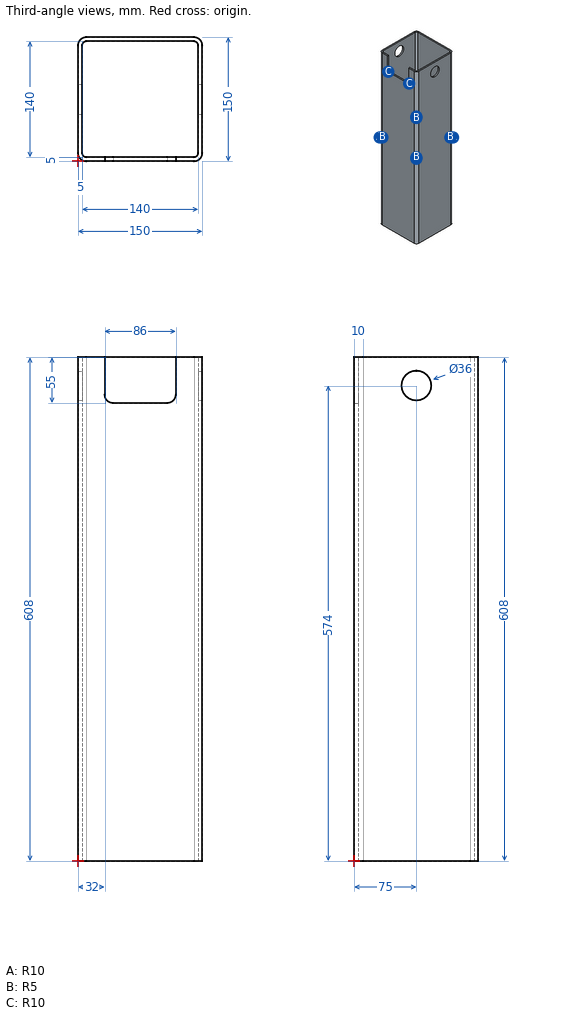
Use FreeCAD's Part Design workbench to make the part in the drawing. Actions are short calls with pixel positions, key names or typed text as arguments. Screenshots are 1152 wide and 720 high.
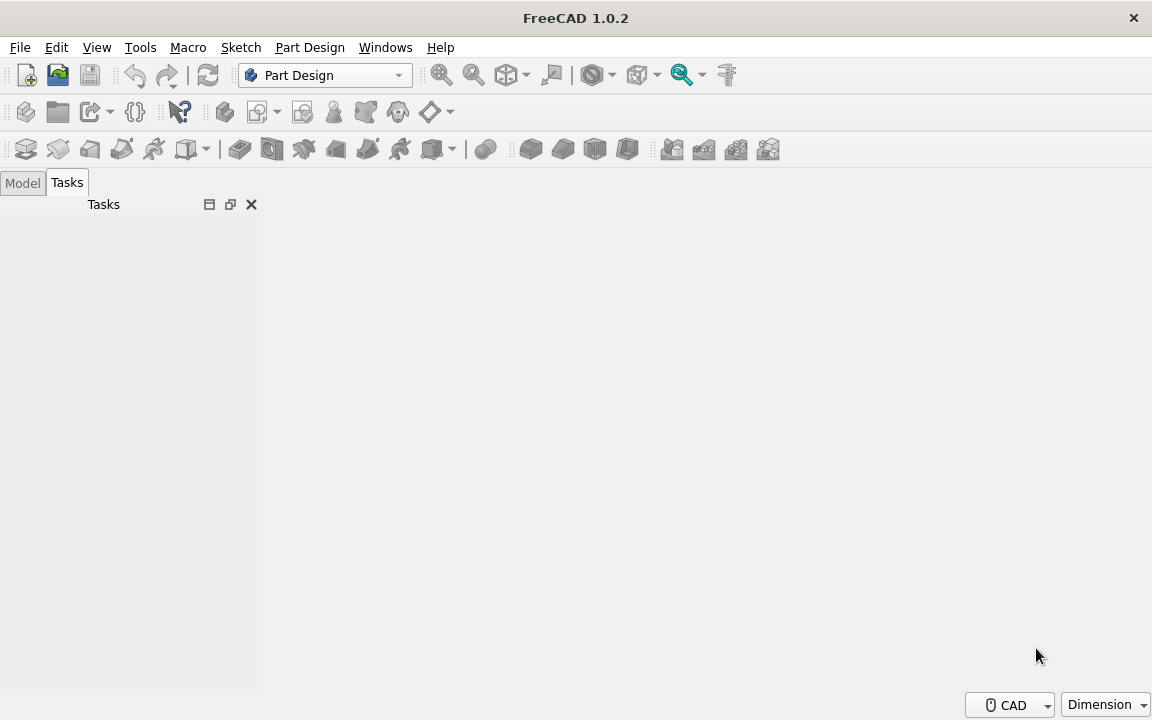
key(ctrl+n)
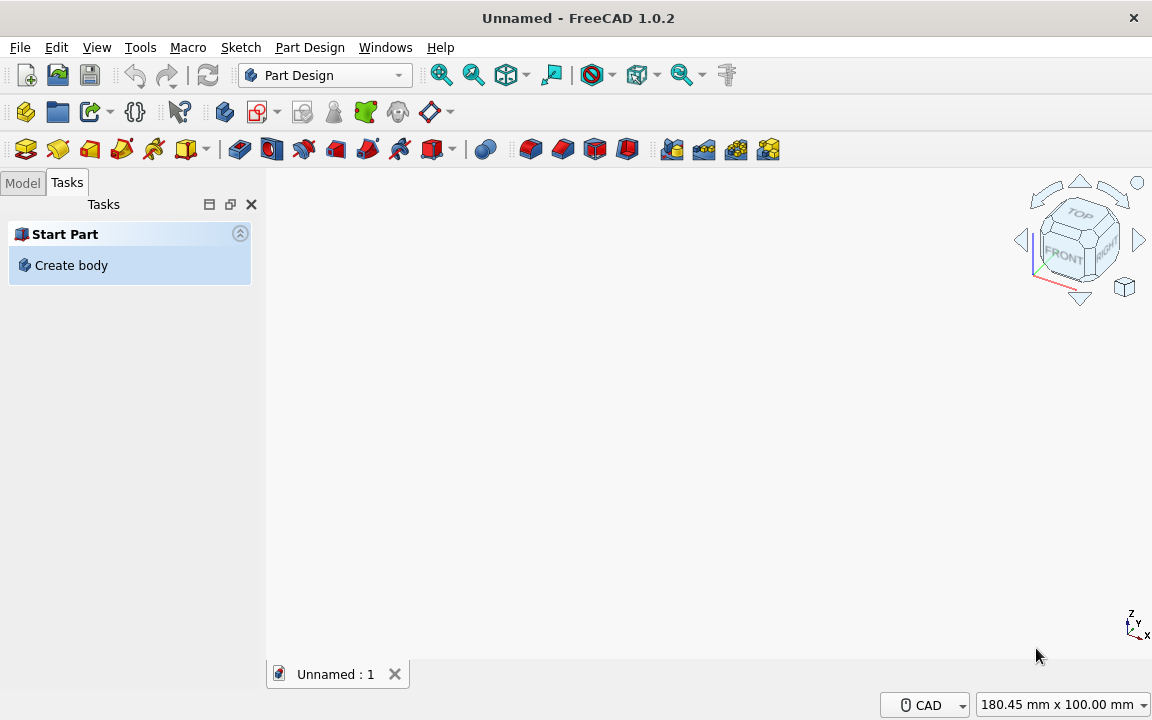
click(258, 112)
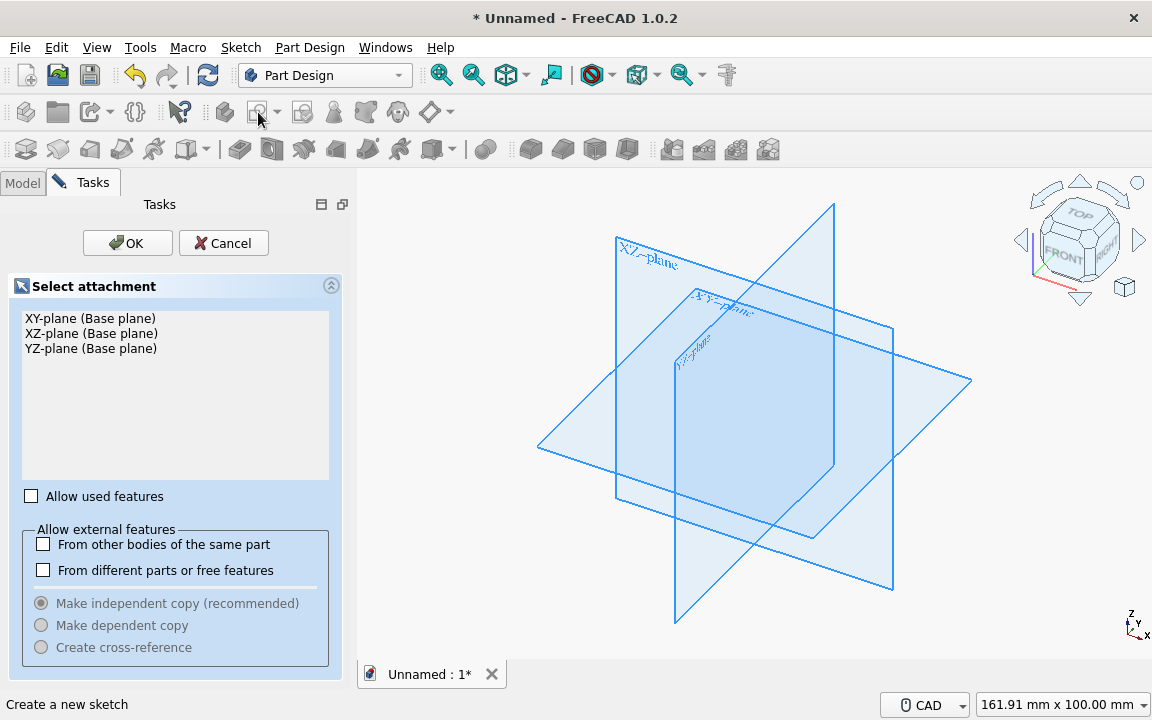
click(82, 318)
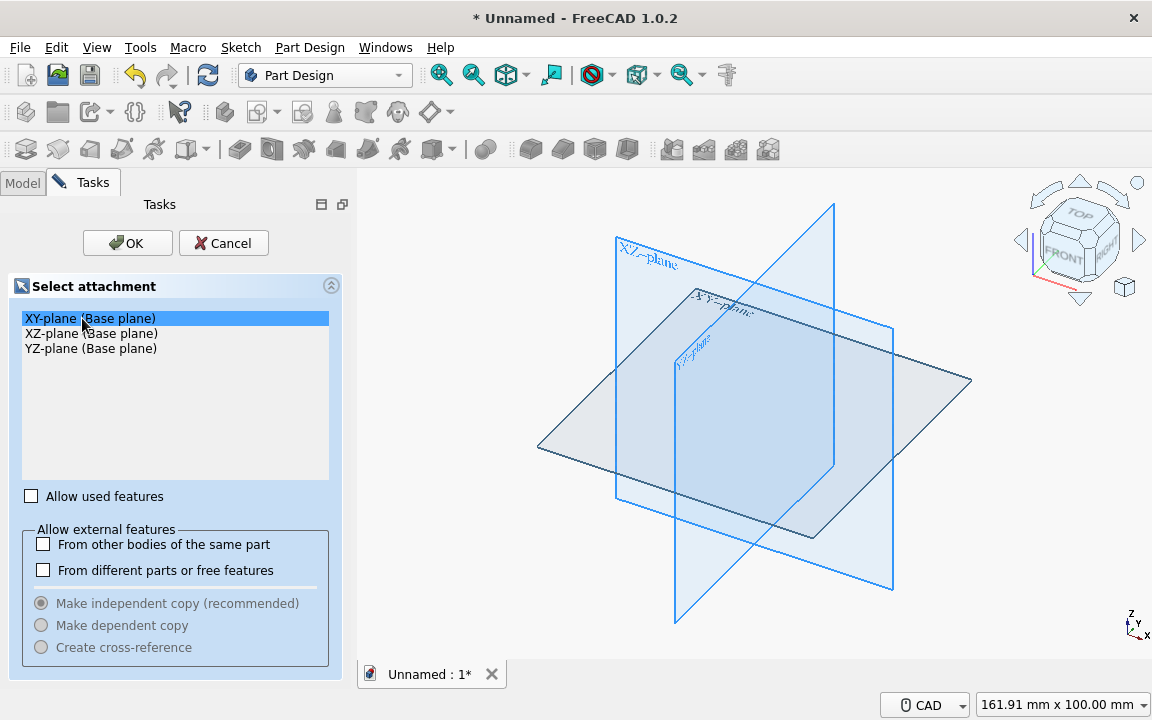
click(128, 243)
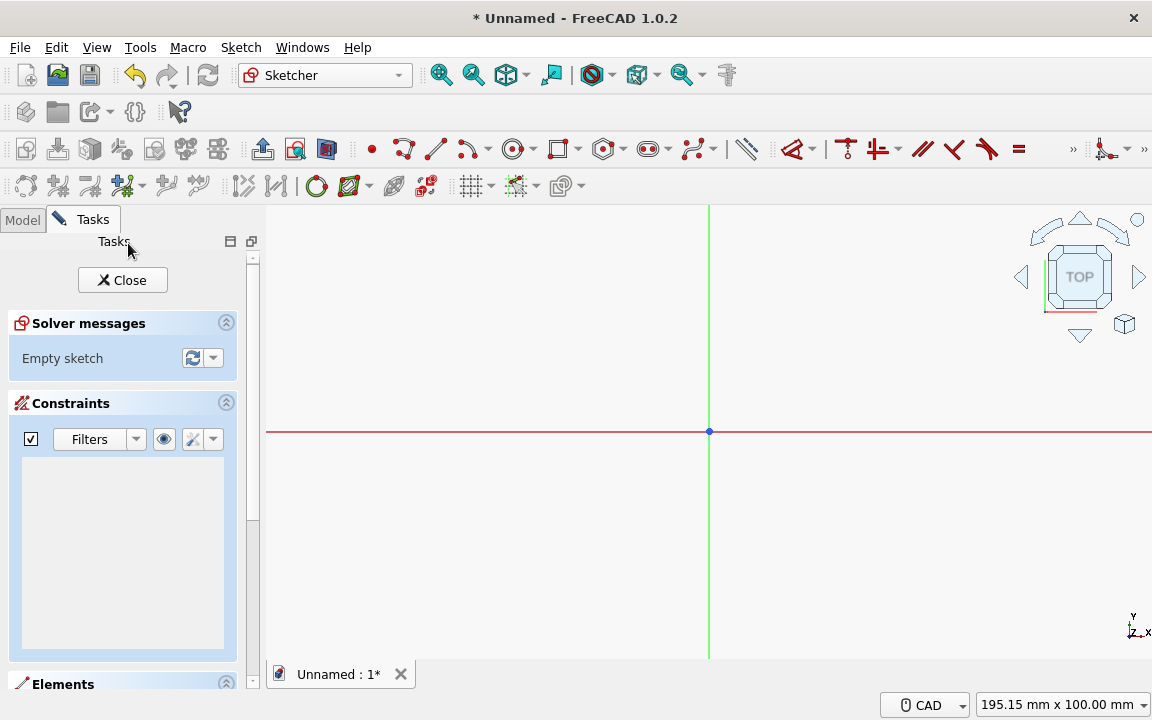
scroll(402, 630, down, 5)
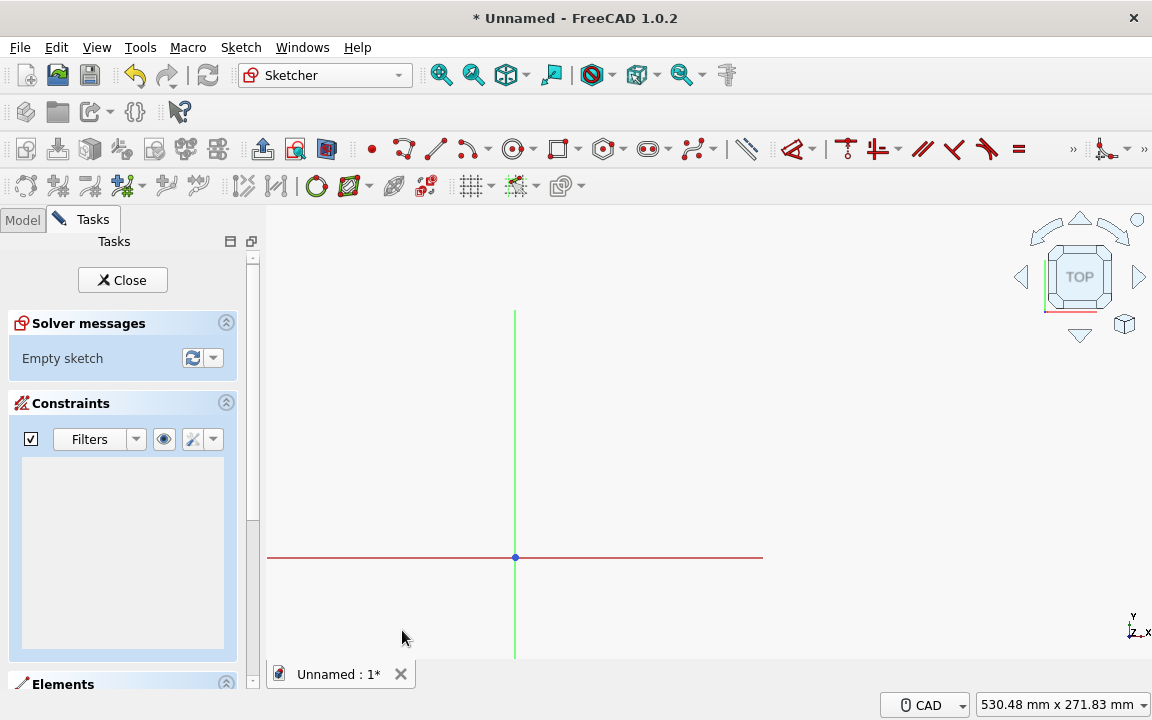
key(g)
key(r)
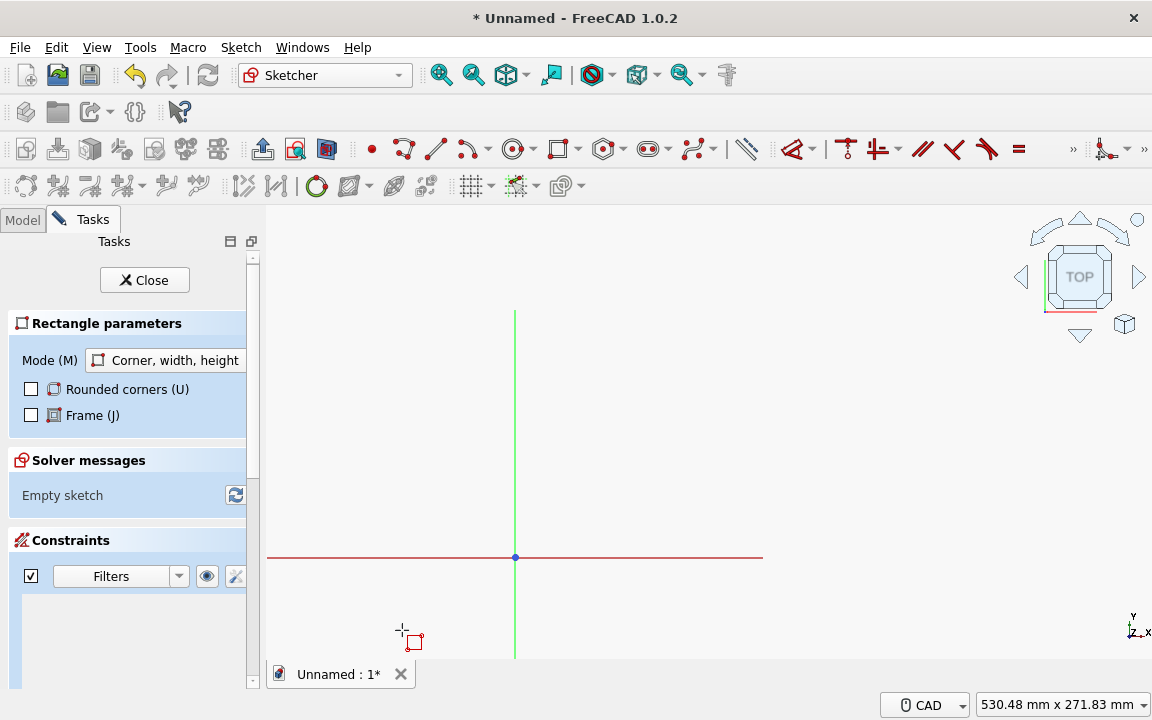
click(515, 558)
click(766, 307)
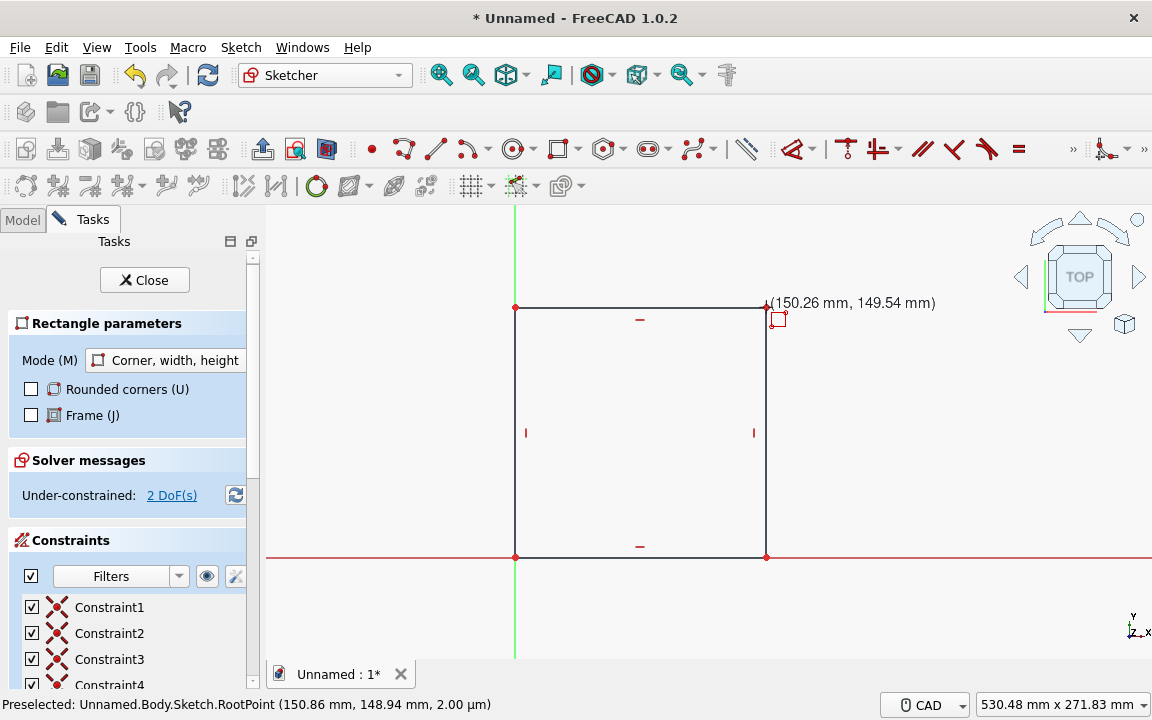
scroll(523, 316, up, 4)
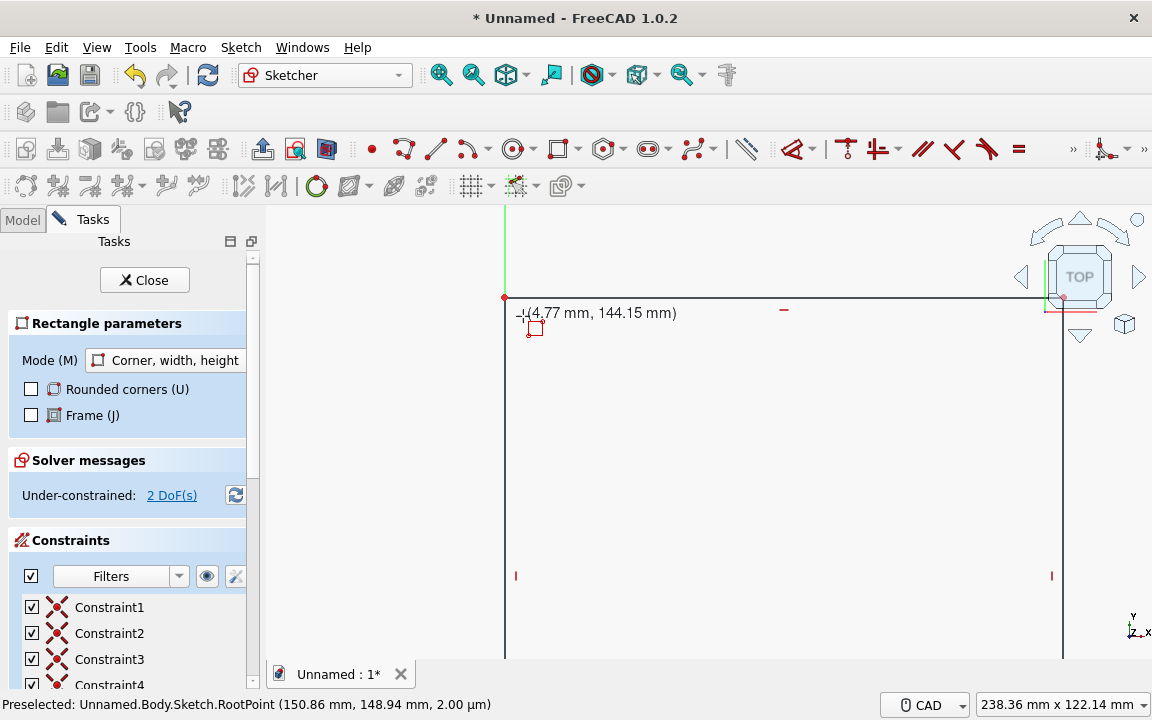
click(524, 315)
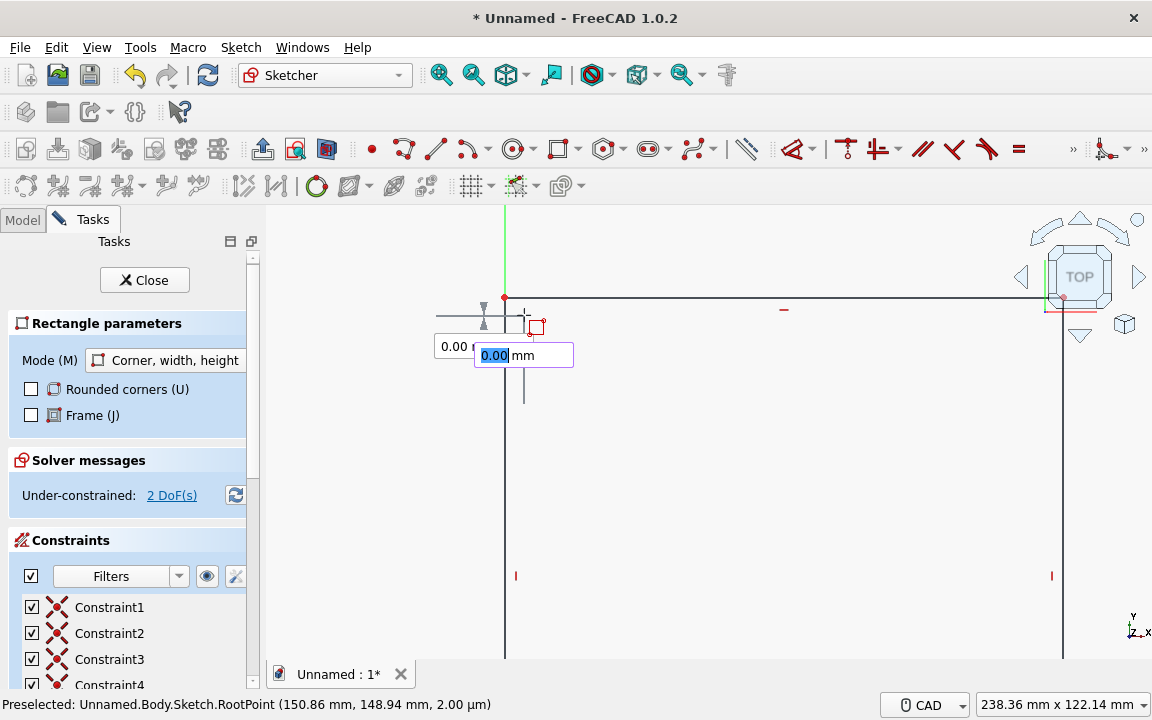
scroll(466, 258, down, 3)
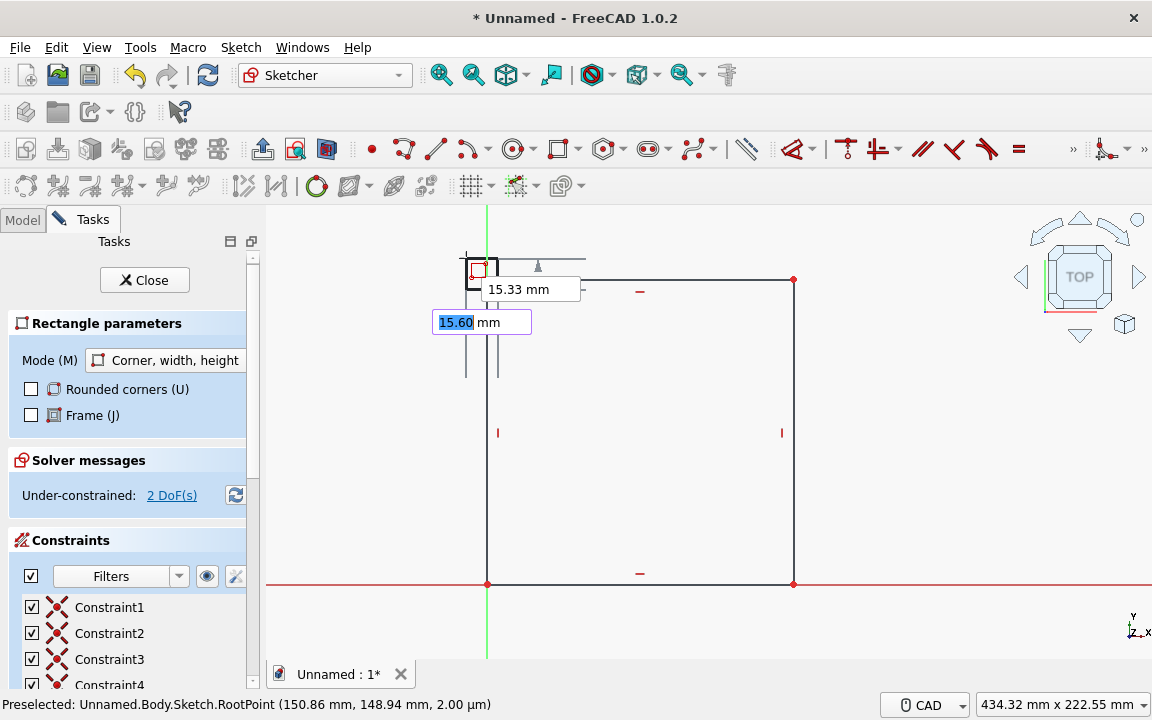
scroll(783, 575, up, 3)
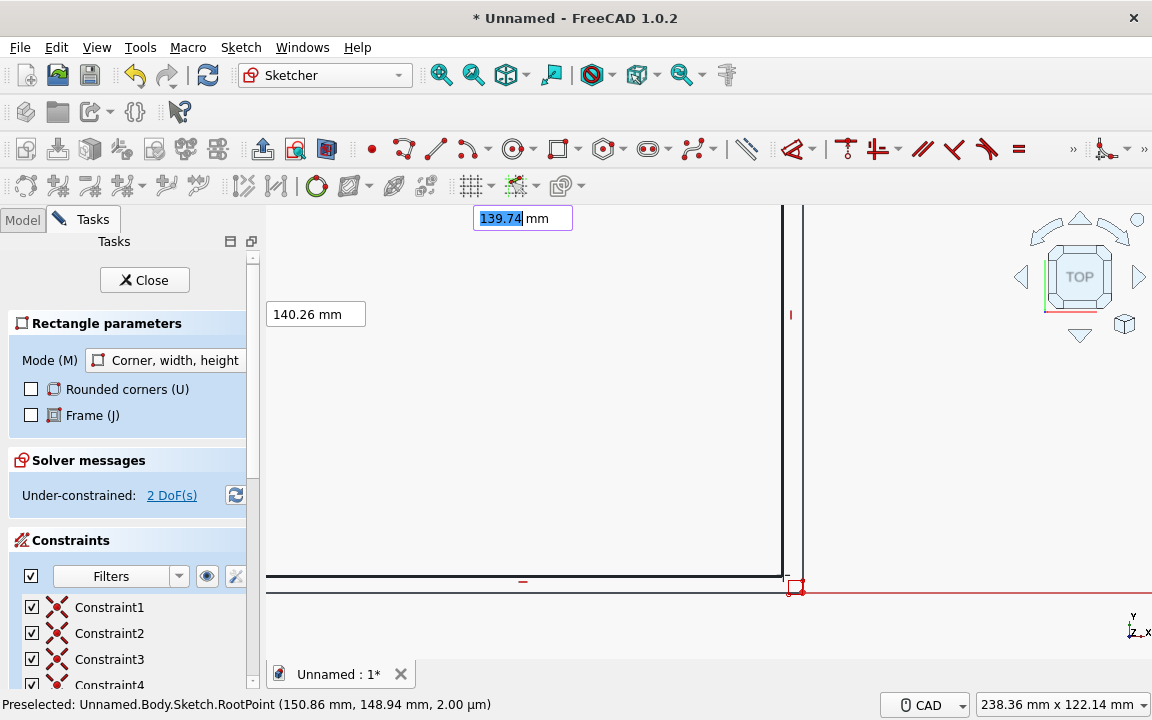
click(783, 574)
key(Escape)